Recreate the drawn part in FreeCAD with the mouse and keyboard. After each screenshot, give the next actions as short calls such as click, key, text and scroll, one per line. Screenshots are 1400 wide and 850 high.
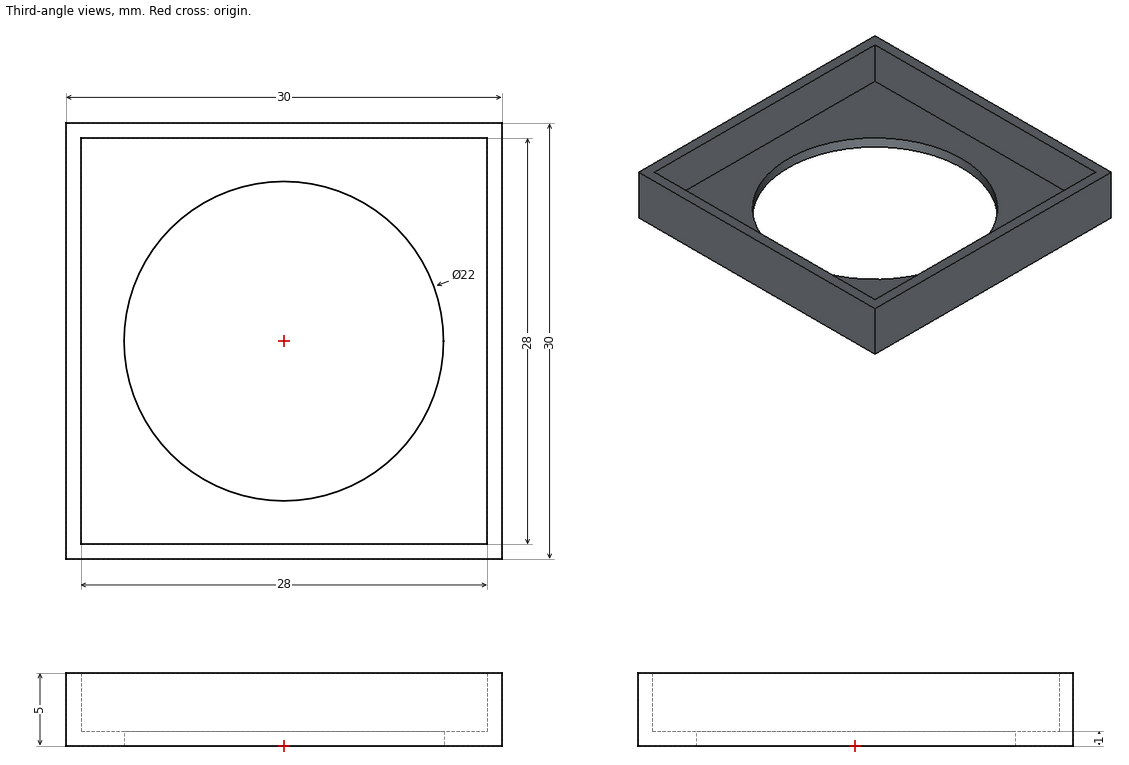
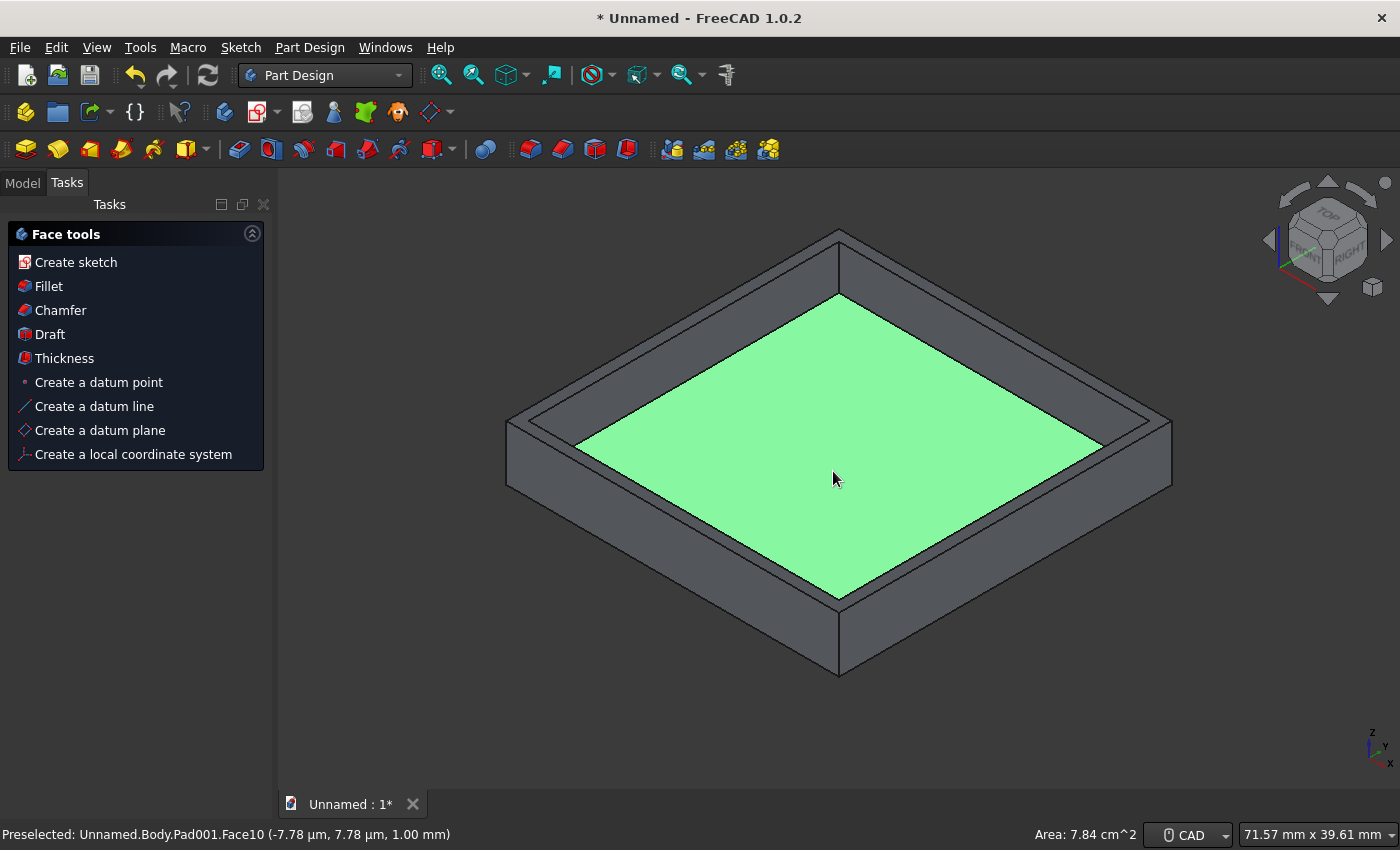
click(258, 112)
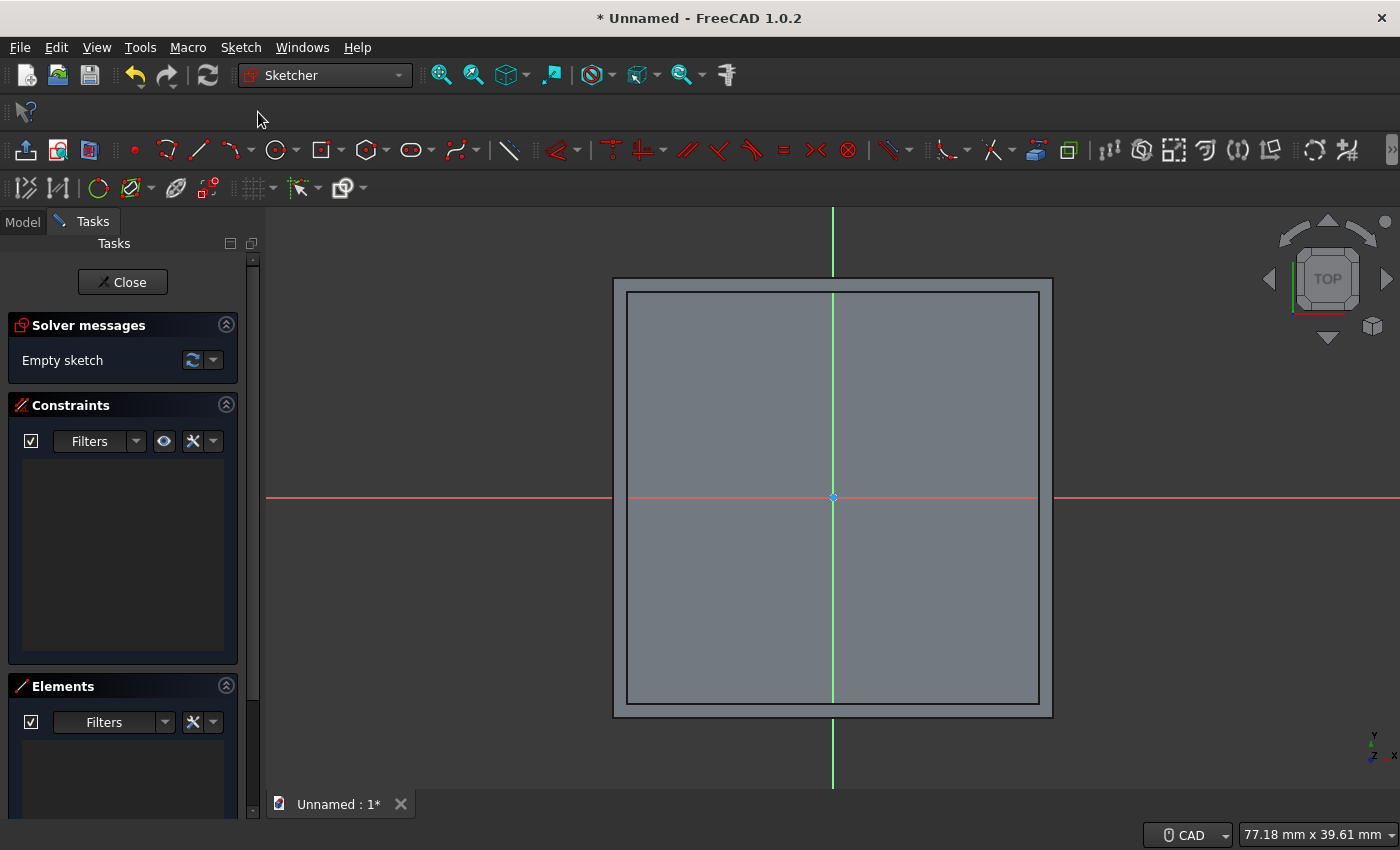
click(276, 150)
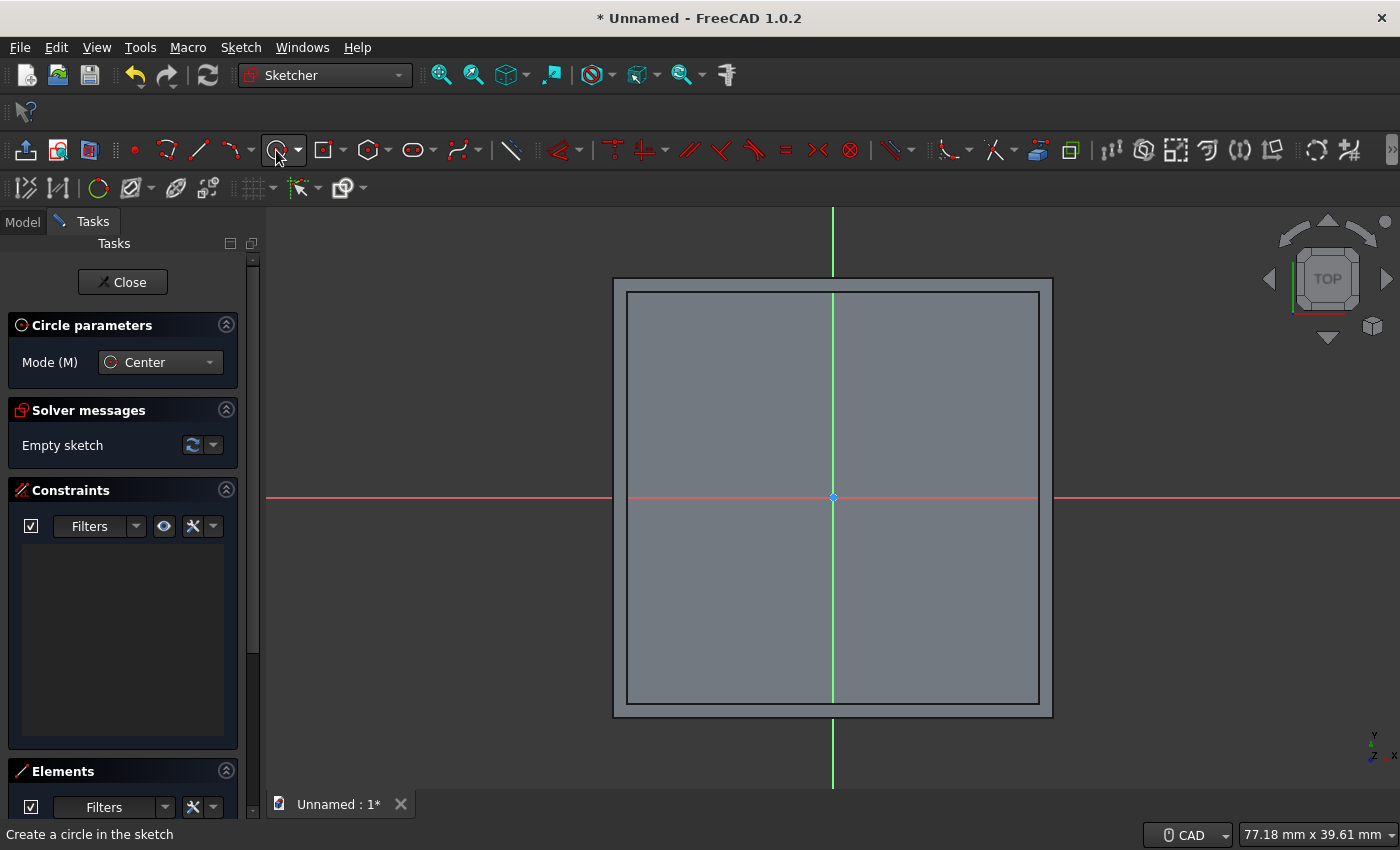
click(833, 498)
click(947, 384)
key(Escape)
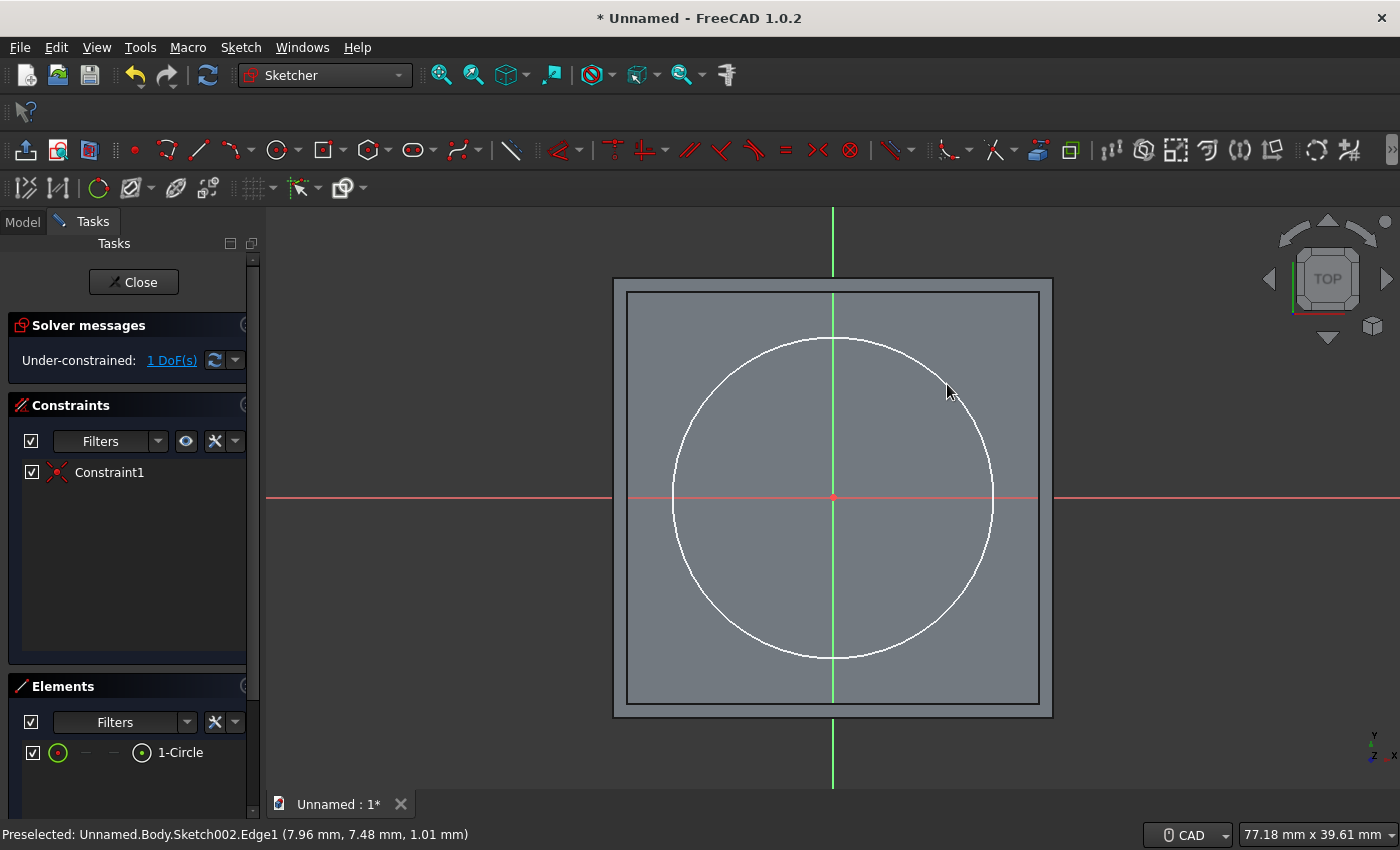
click(558, 150)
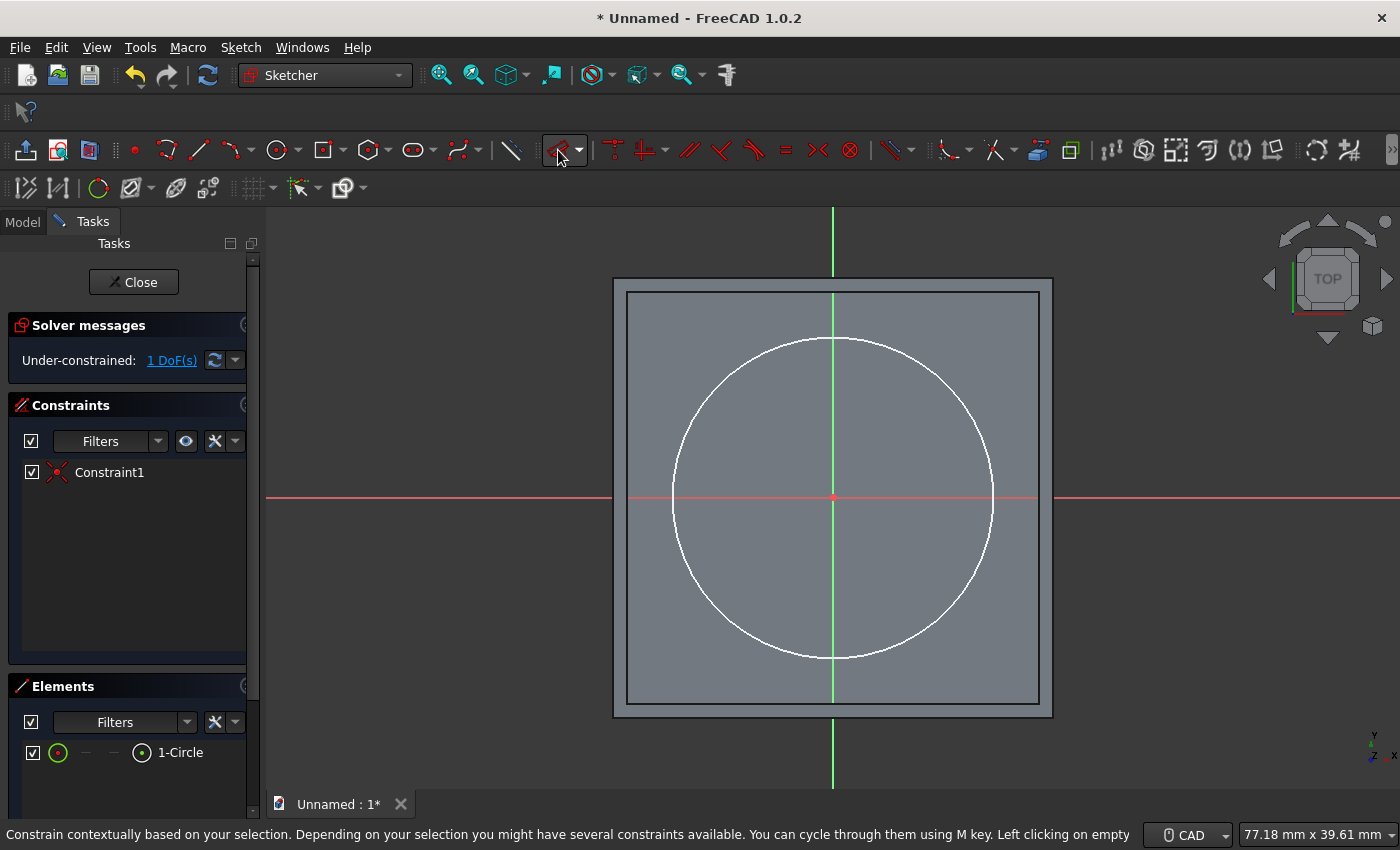
click(946, 384)
click(969, 361)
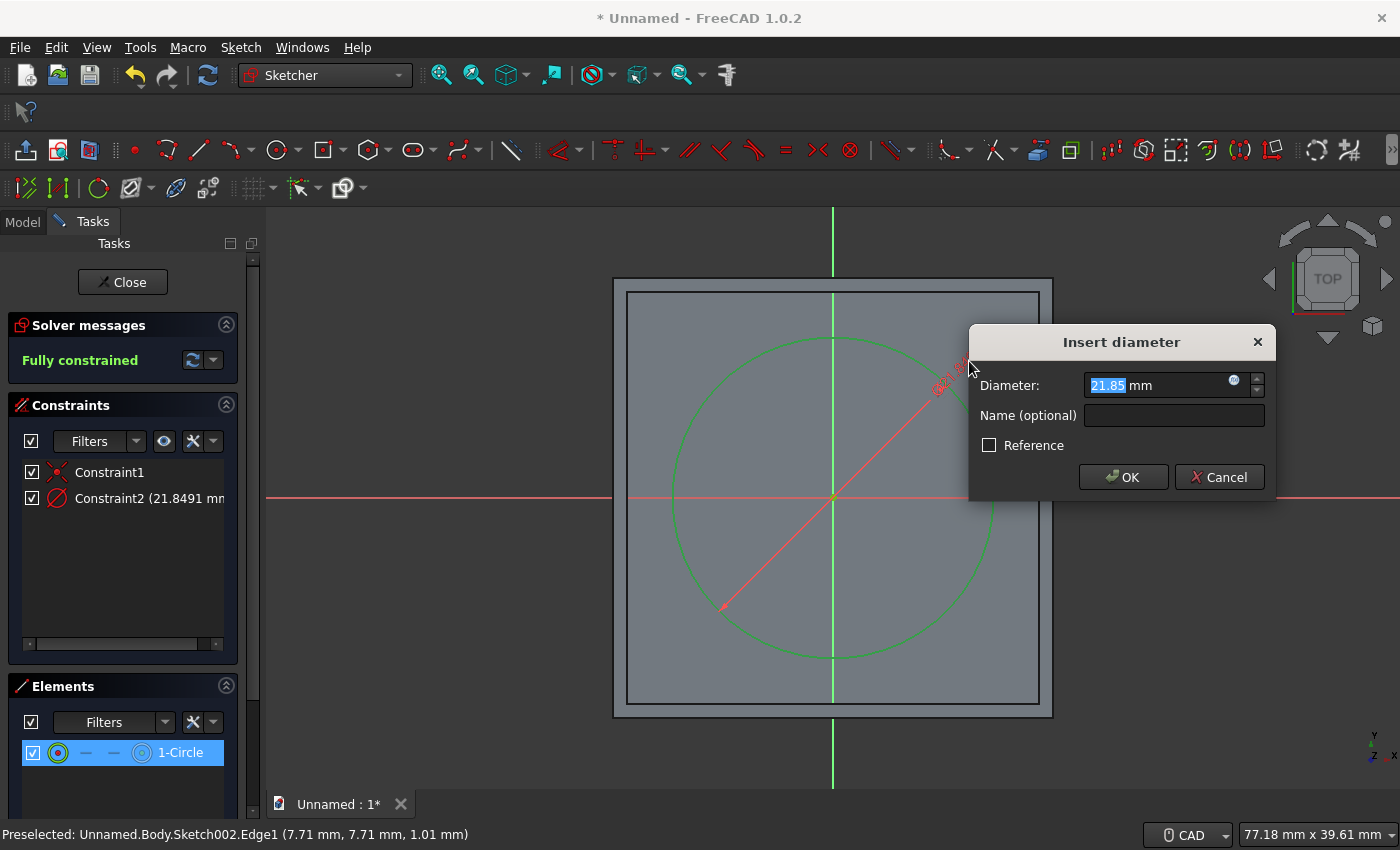
text(22)
key(Return)
key(Escape)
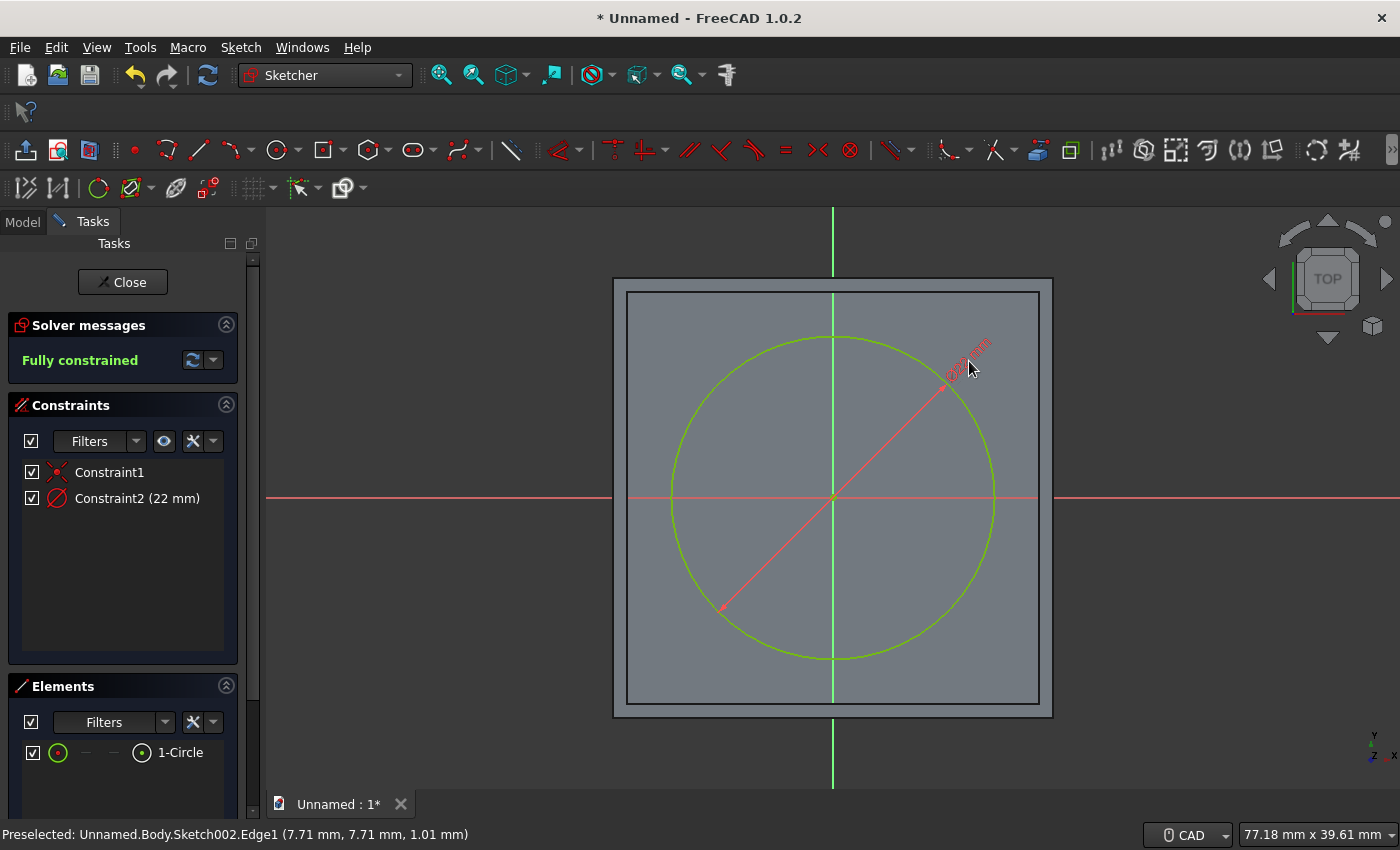
click(123, 282)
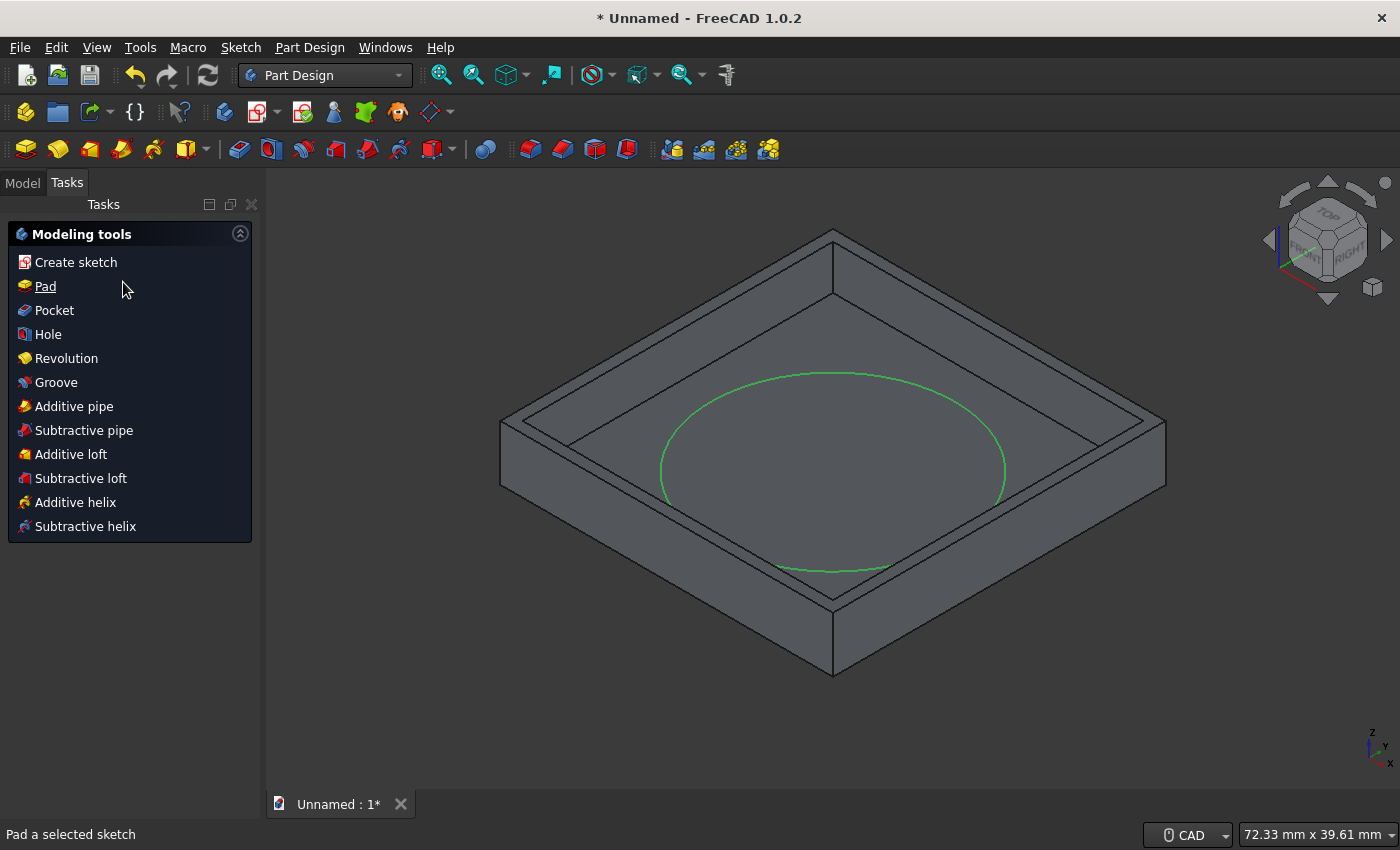
click(240, 150)